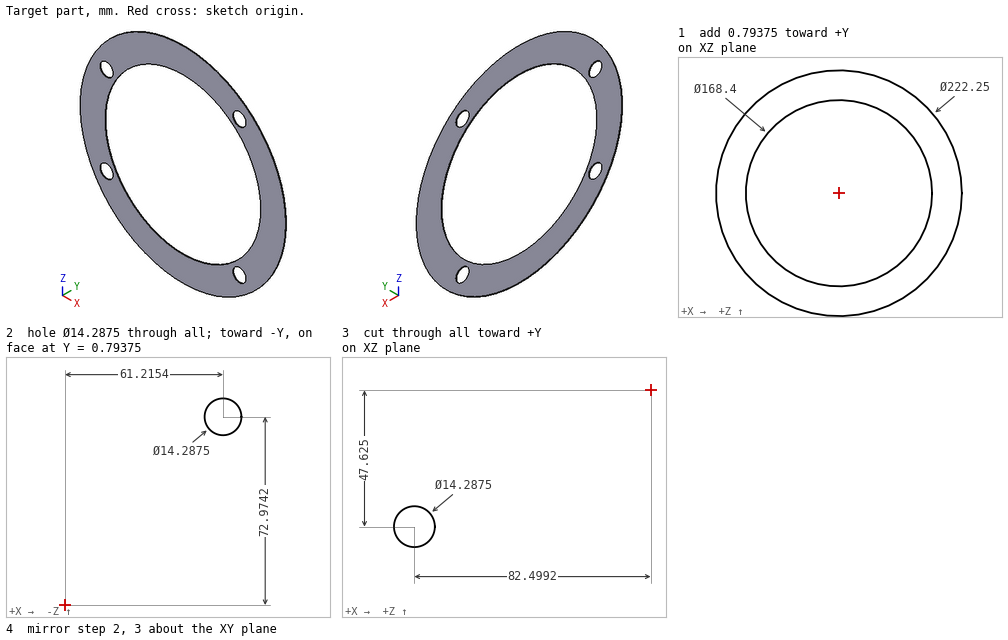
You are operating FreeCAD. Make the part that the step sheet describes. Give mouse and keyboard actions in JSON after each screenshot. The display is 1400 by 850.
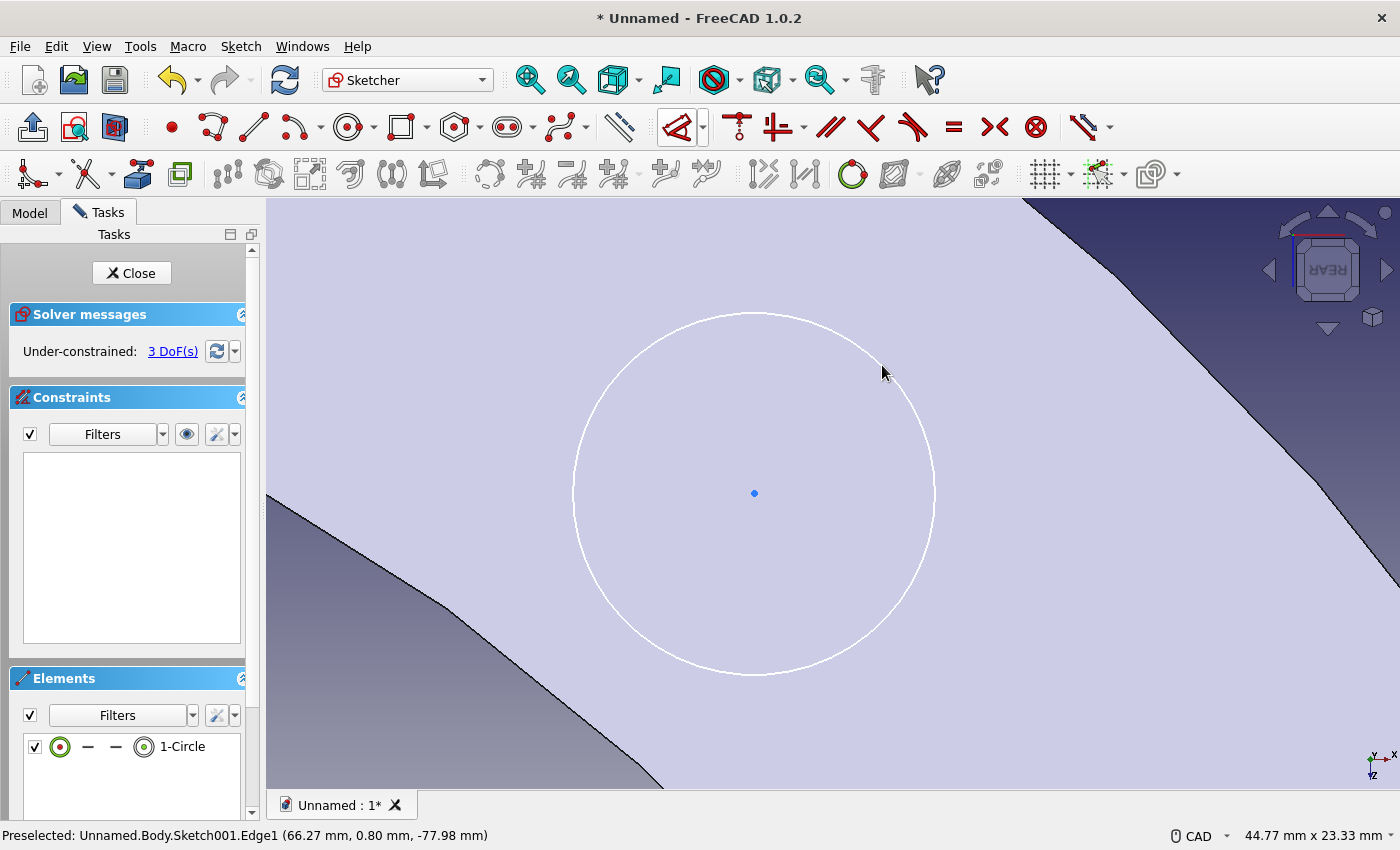
{"action": "left_click", "coordinate": [882, 366]}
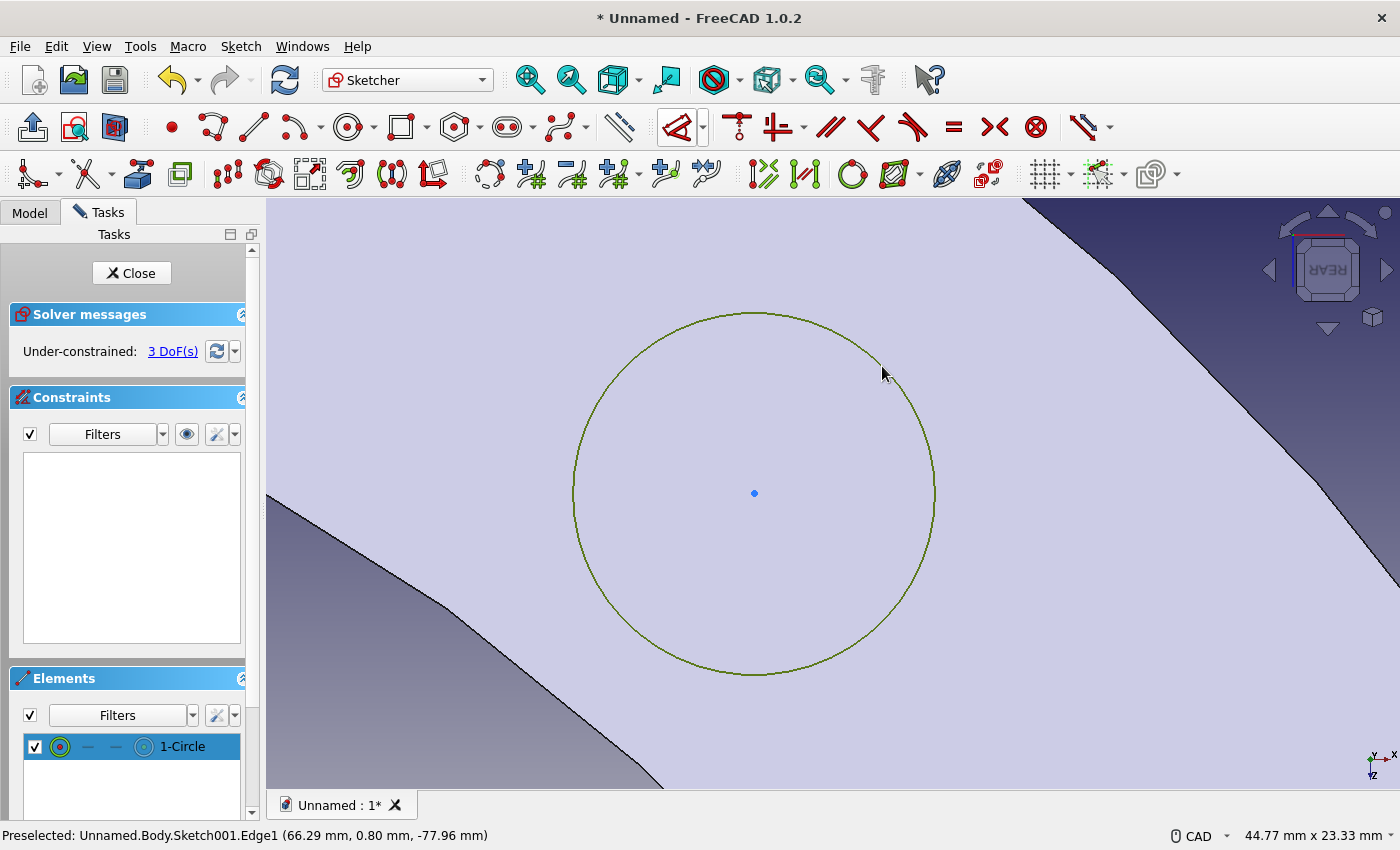
{"action": "key", "text": "k o"}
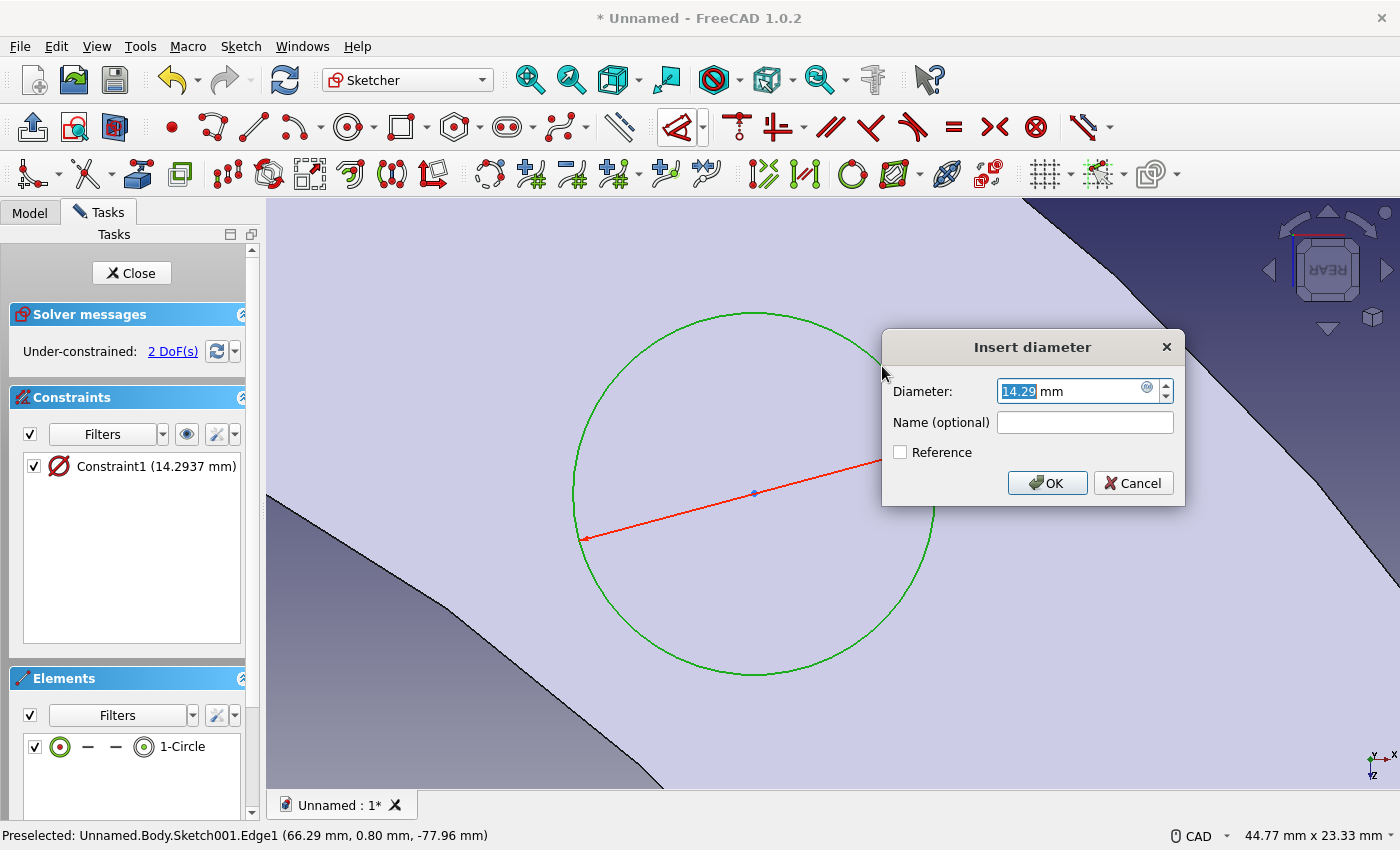
{"action": "type", "text": "14.2875"}
{"action": "key", "text": "Return"}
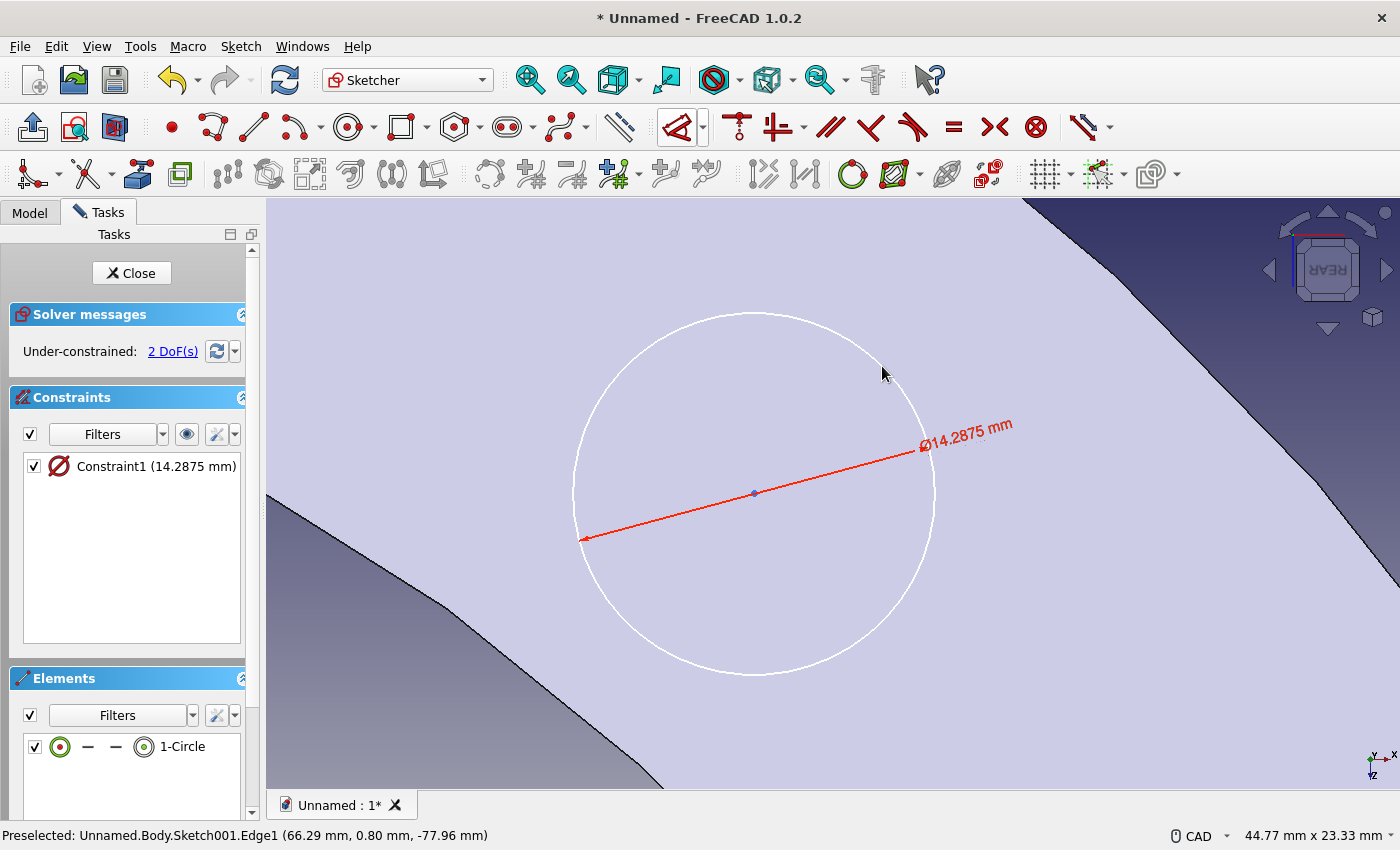
{"action": "left_click", "coordinate": [754, 494]}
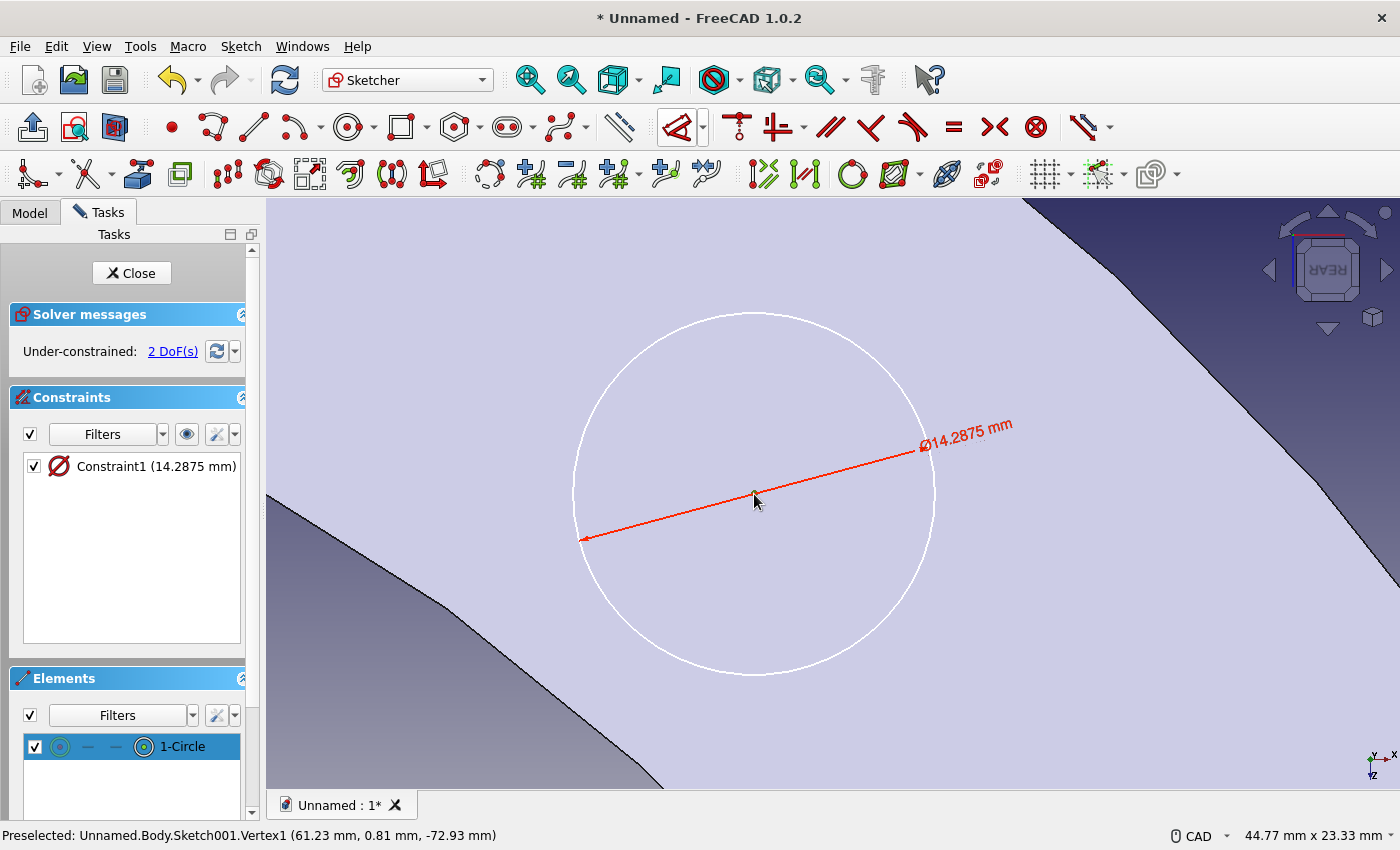
{"action": "left_click", "coordinate": [702, 128]}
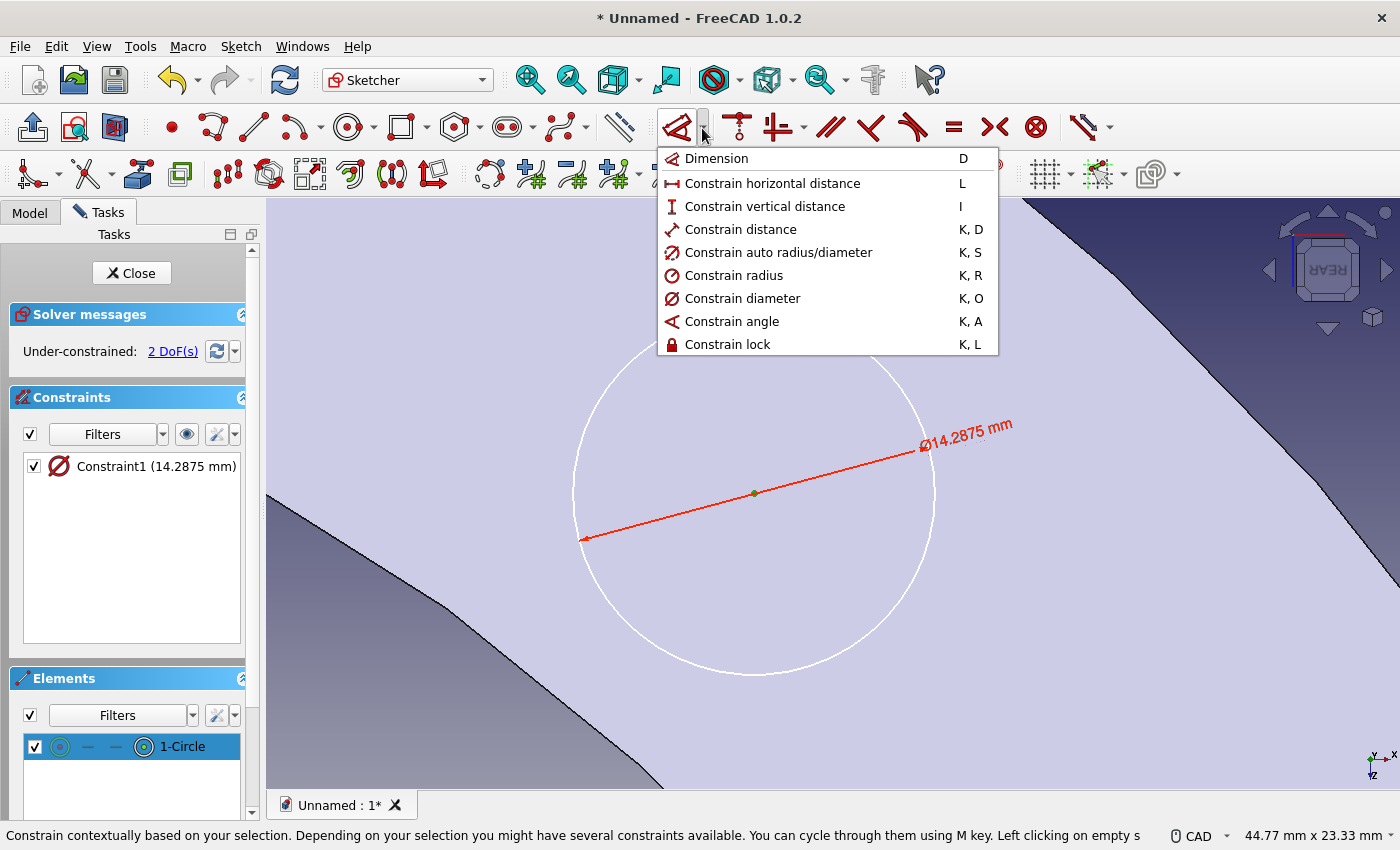
{"action": "left_click", "coordinate": [828, 184]}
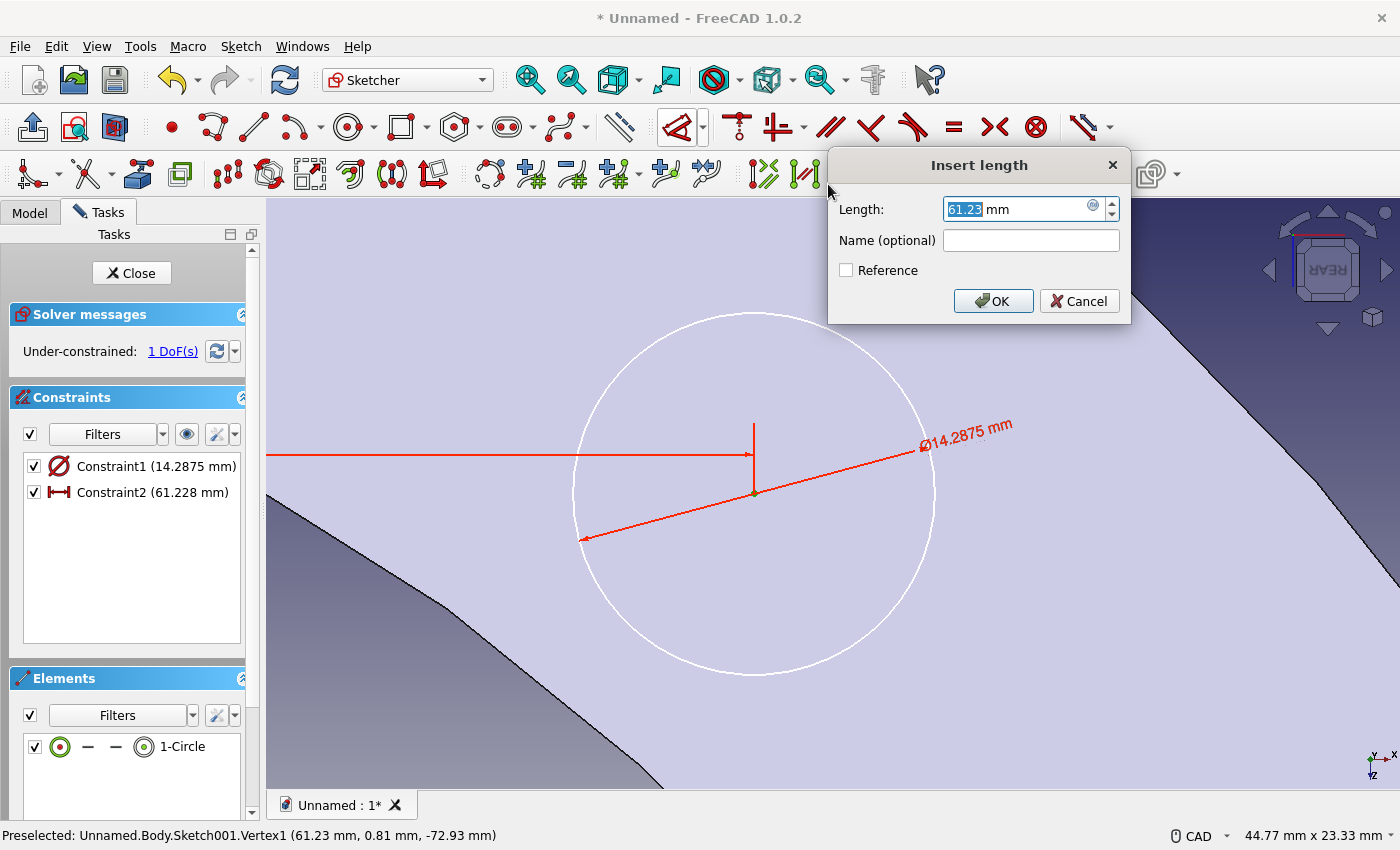
{"action": "type", "text": "61.2154"}
{"action": "key", "text": "Return"}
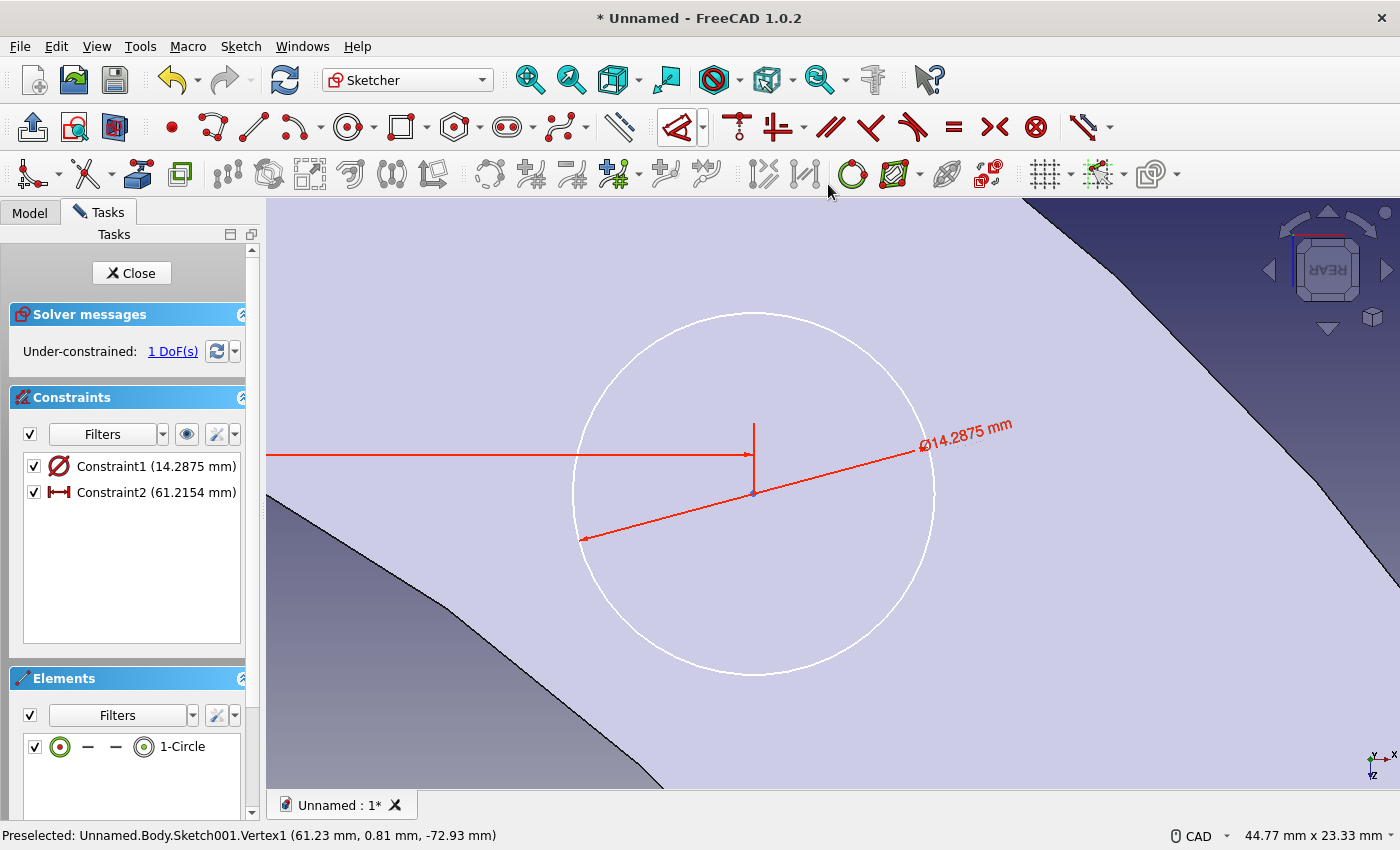
{"action": "left_click", "coordinate": [754, 494]}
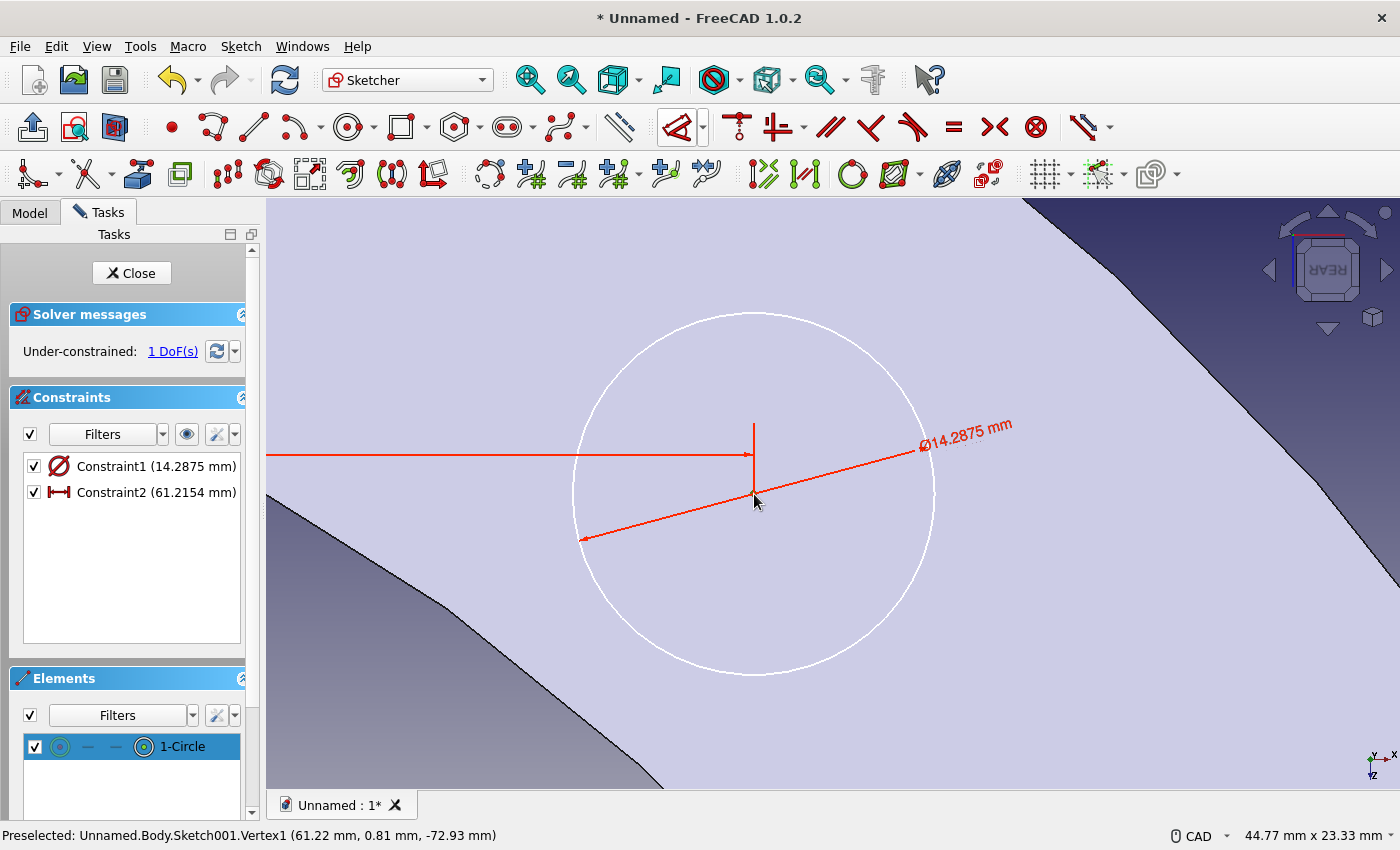
{"action": "key", "text": "i"}